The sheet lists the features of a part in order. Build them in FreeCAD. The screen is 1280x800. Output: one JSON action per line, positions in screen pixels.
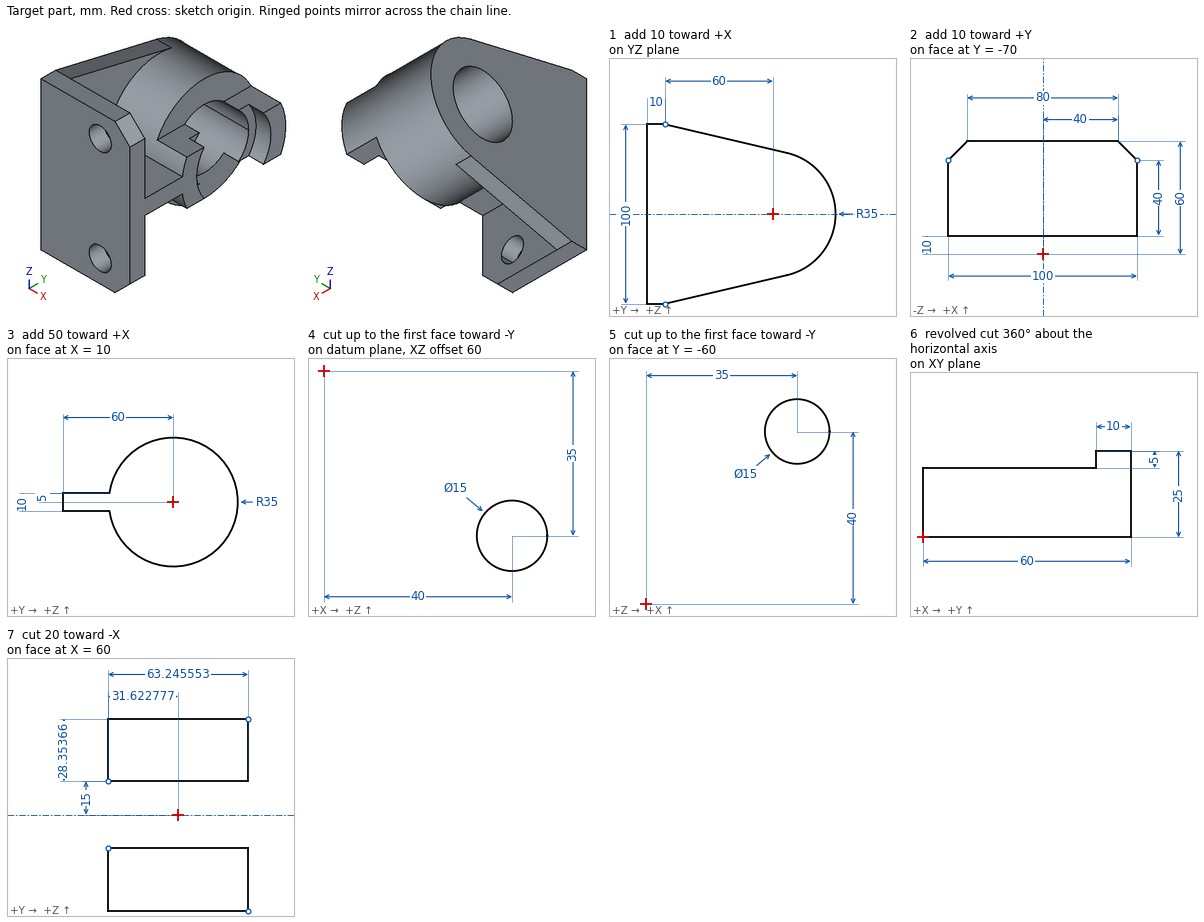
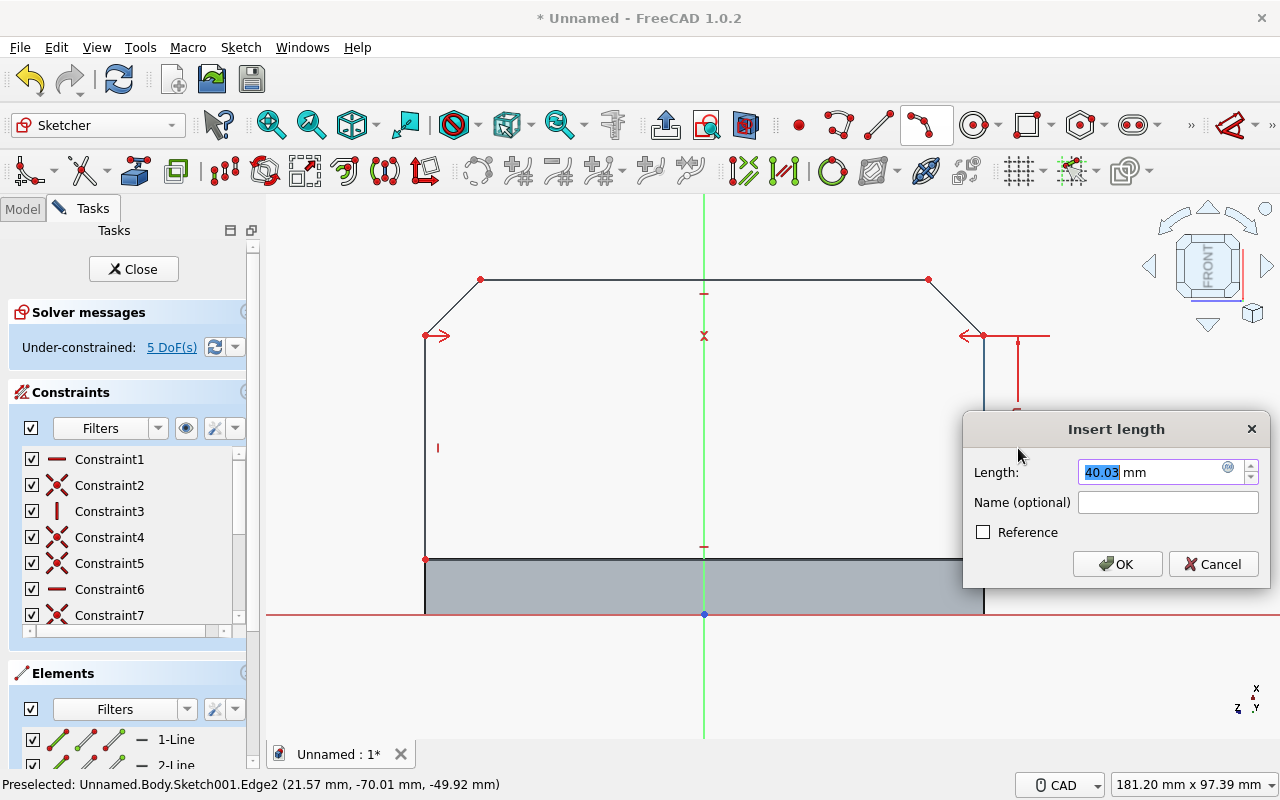
{"action": "type", "text": "40"}
{"action": "key", "text": "Return"}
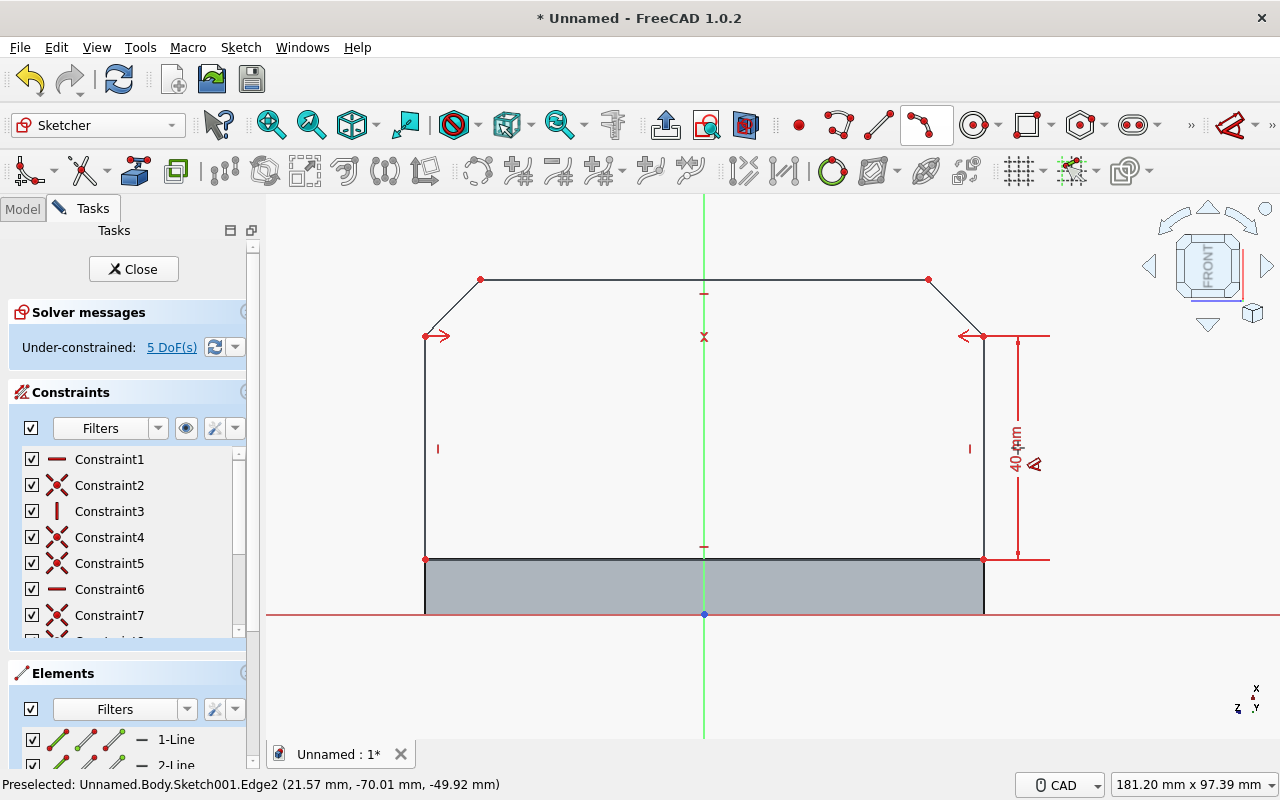
{"action": "left_click", "coordinate": [794, 280]}
{"action": "left_click", "coordinate": [601, 246]}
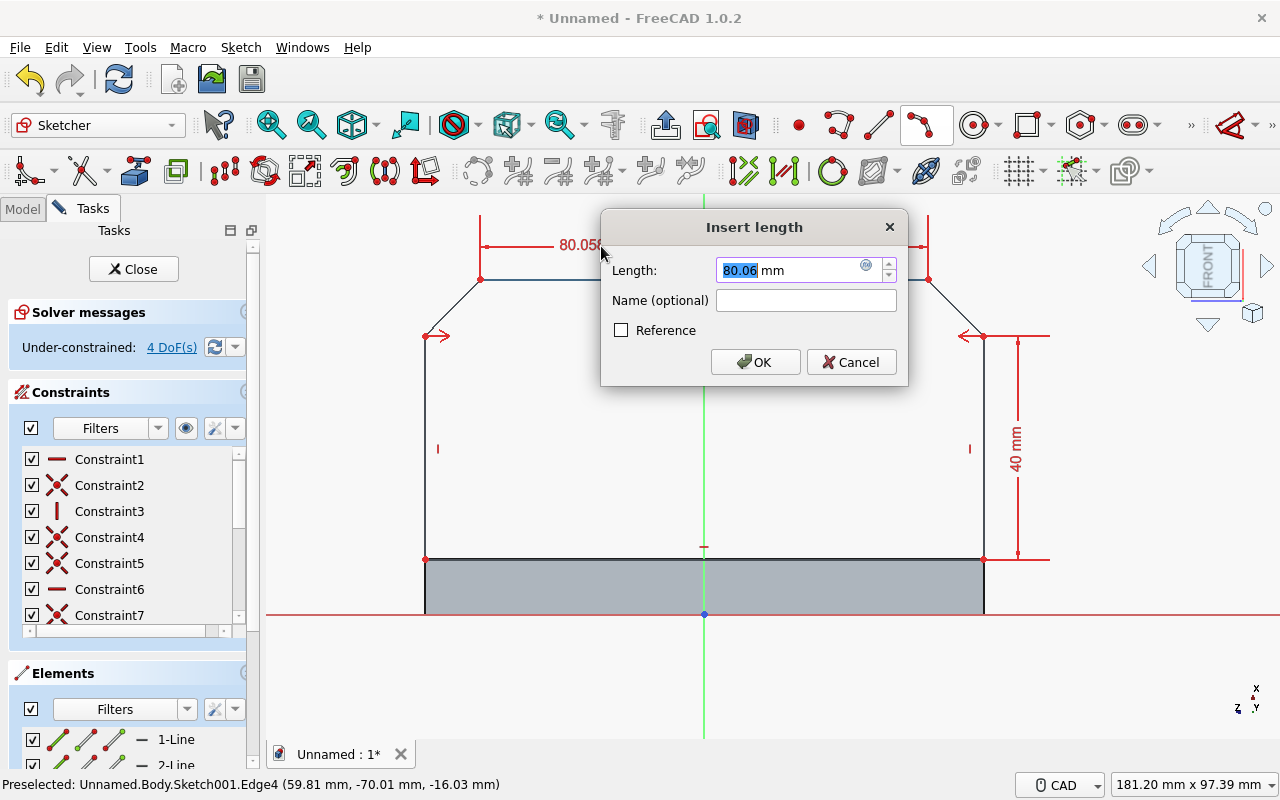
{"action": "type", "text": "80"}
{"action": "key", "text": "Return"}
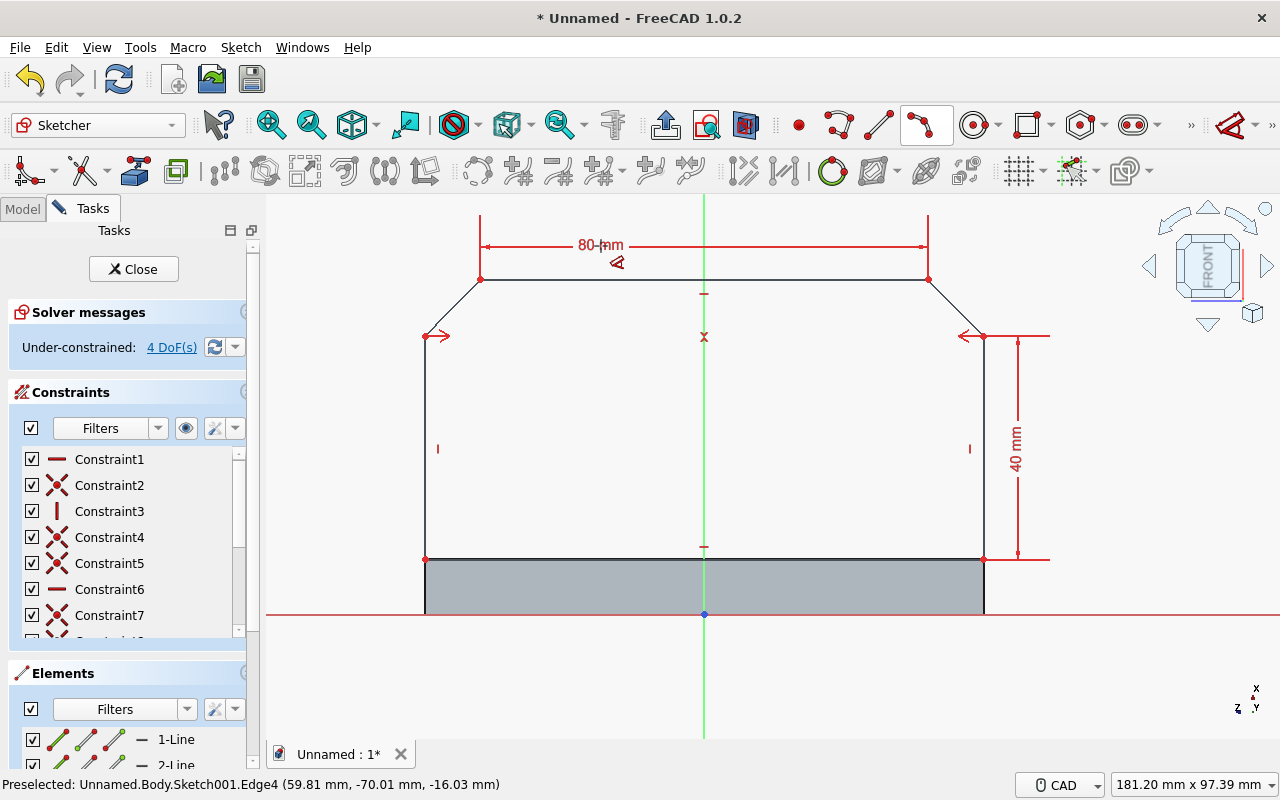
{"action": "left_click", "coordinate": [593, 560]}
{"action": "left_click", "coordinate": [576, 594]}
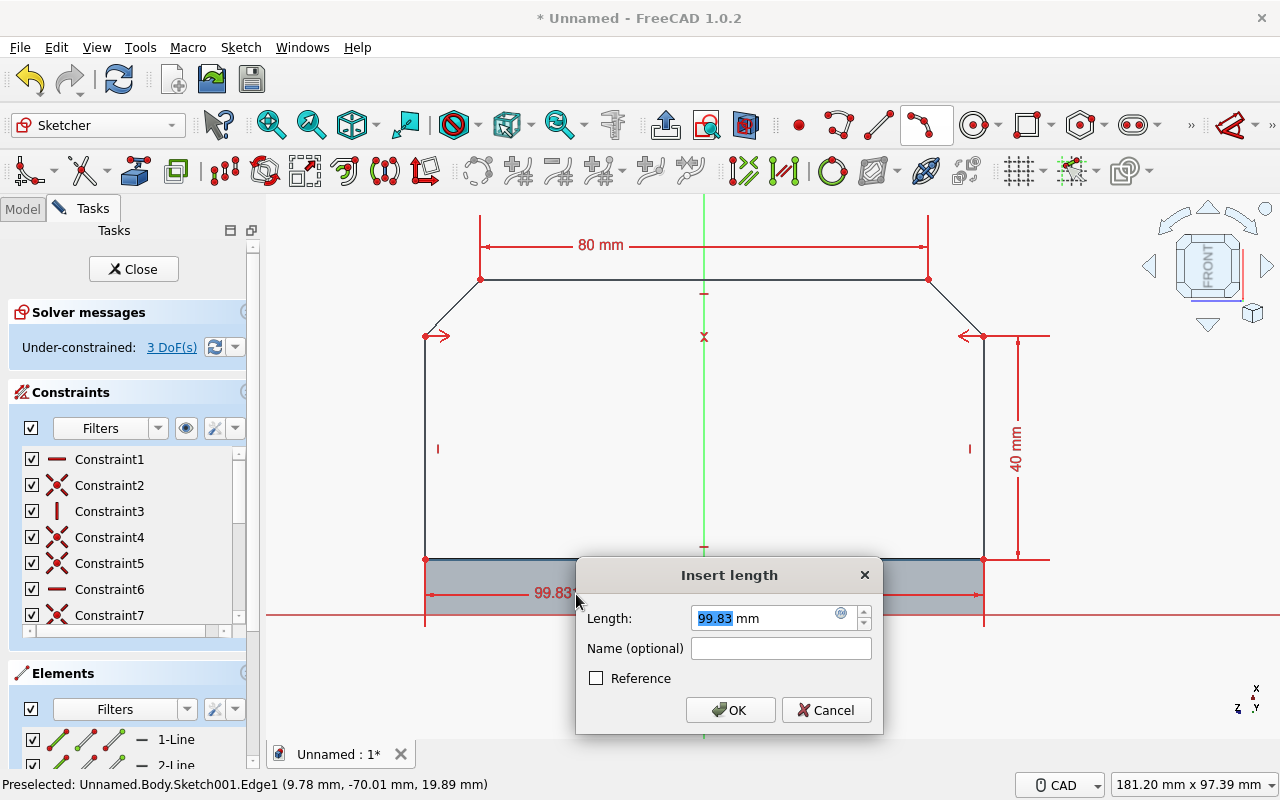
{"action": "type", "text": "100"}
{"action": "key", "text": "Return"}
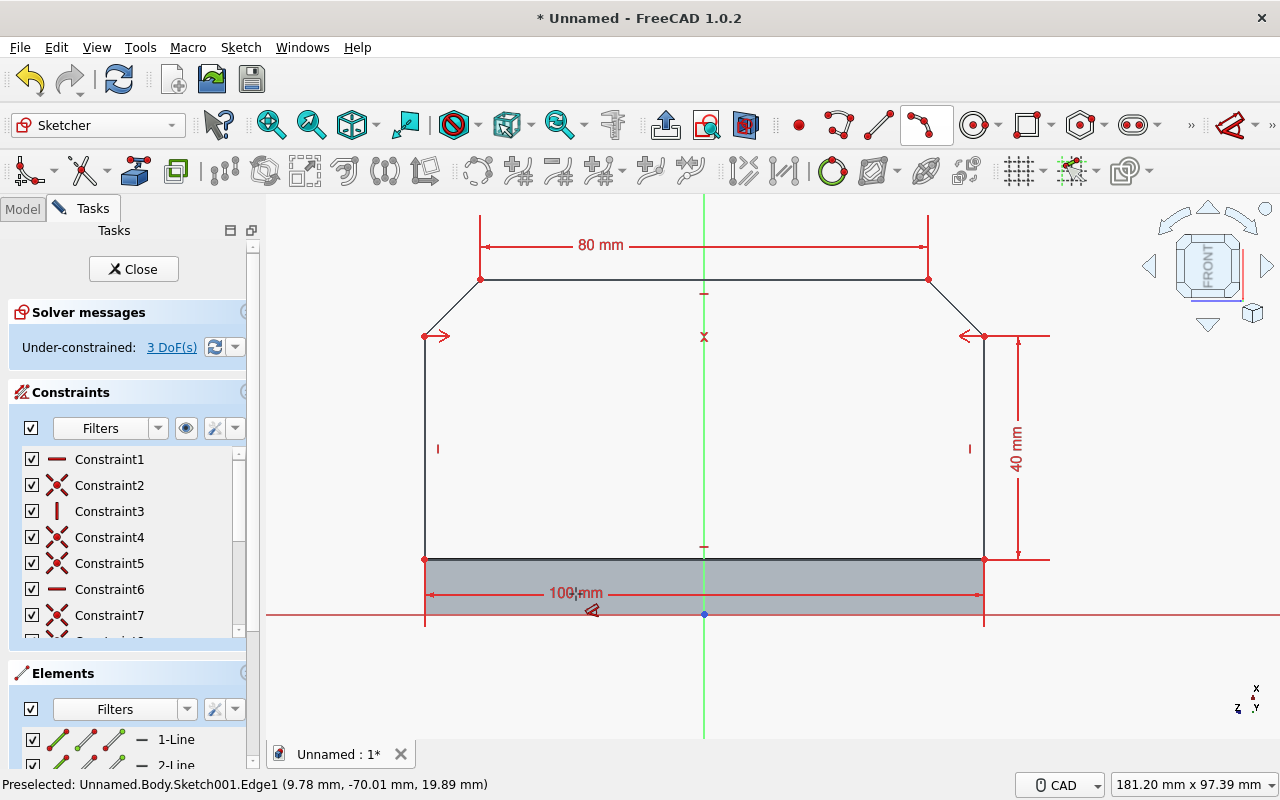
{"action": "left_click", "coordinate": [425, 560]}
{"action": "left_click", "coordinate": [391, 587]}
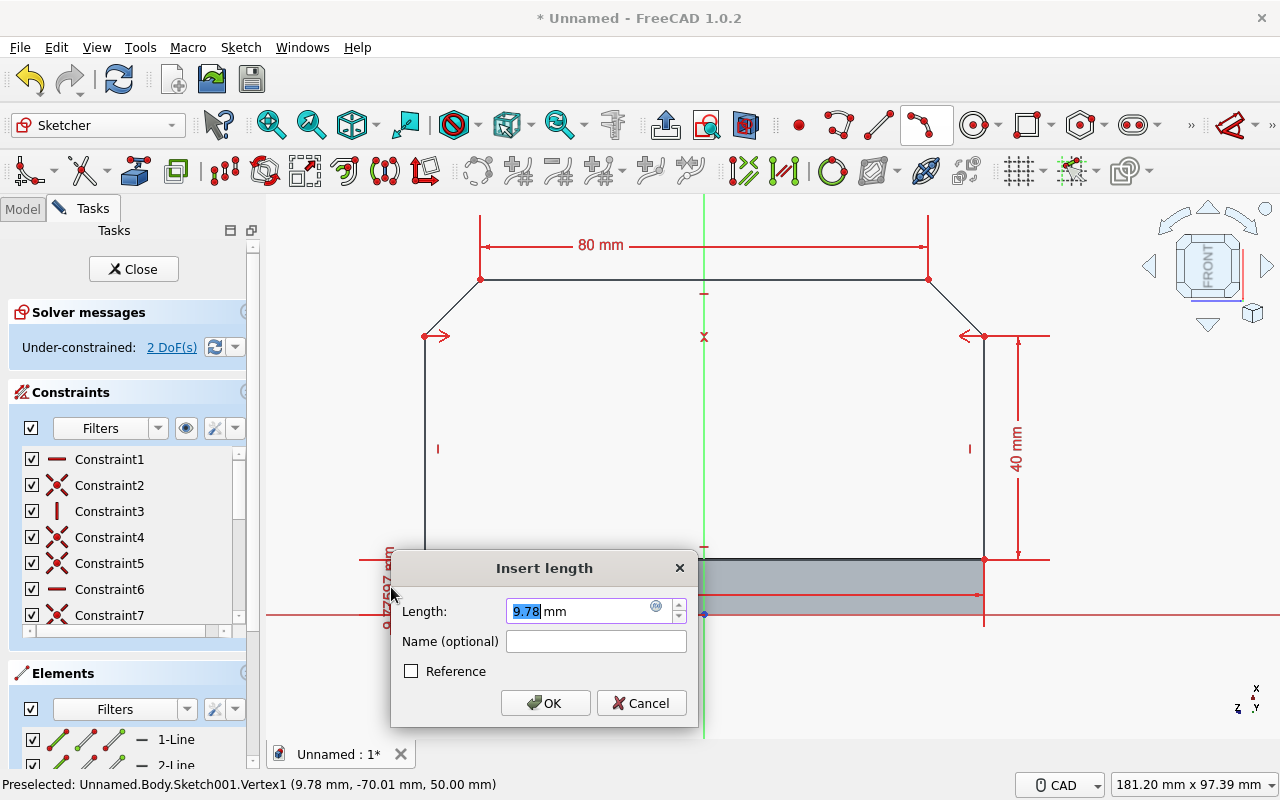
{"action": "type", "text": "10"}
{"action": "key", "text": "Return"}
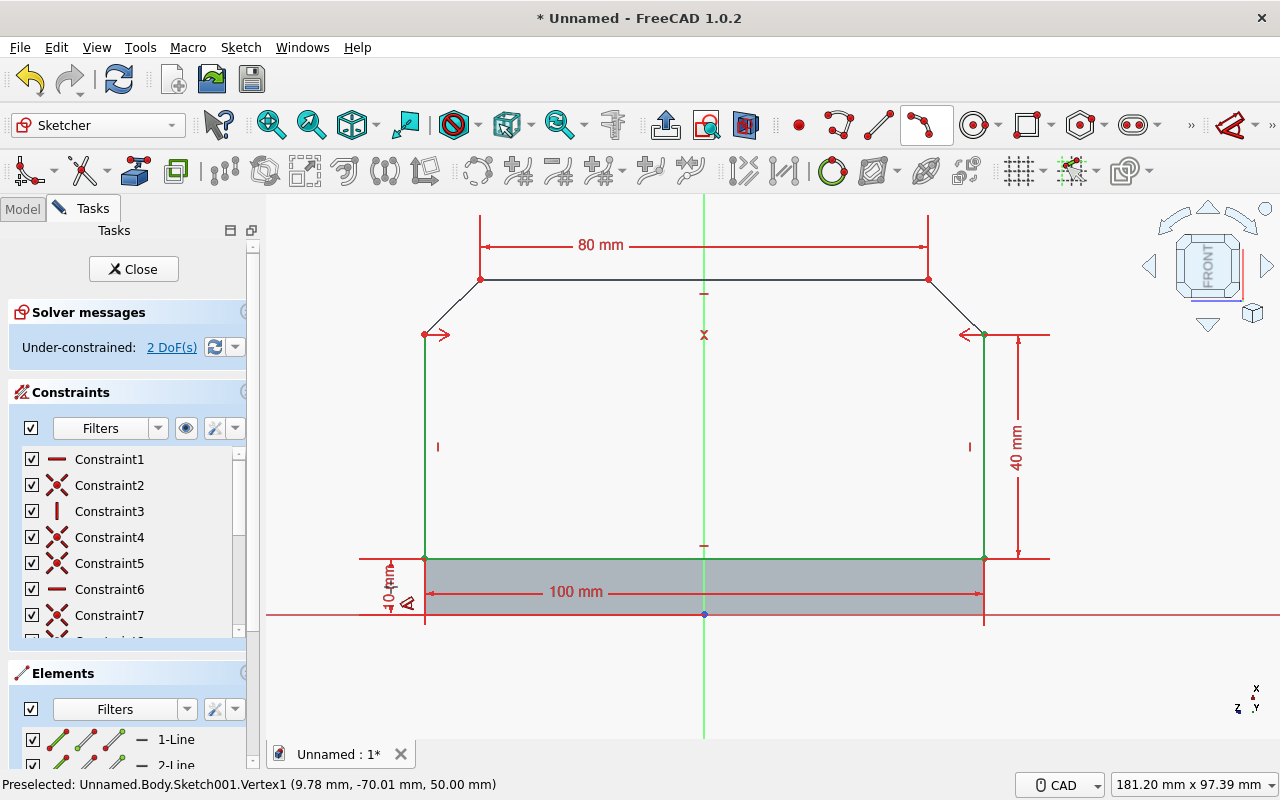
{"action": "left_click", "coordinate": [928, 280]}
{"action": "left_click", "coordinate": [816, 649]}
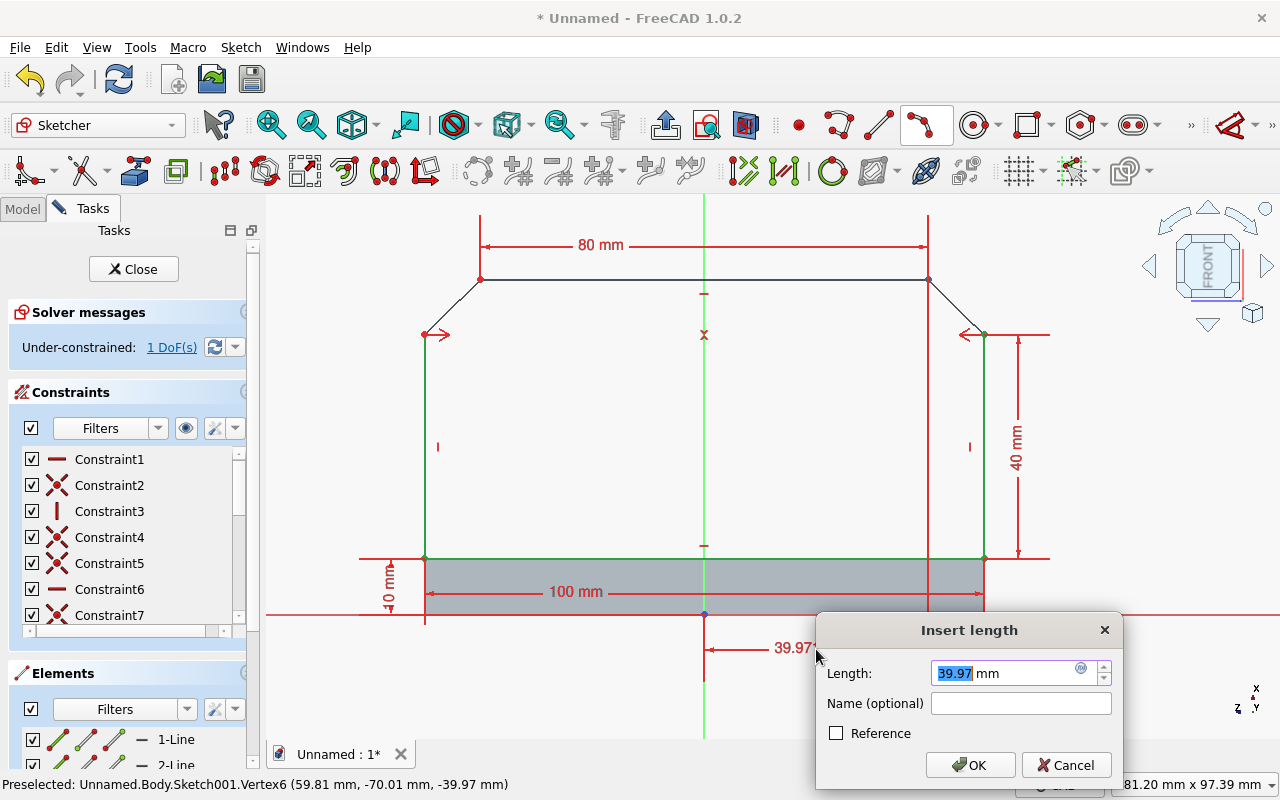
{"action": "type", "text": "40"}
{"action": "key", "text": "Return"}